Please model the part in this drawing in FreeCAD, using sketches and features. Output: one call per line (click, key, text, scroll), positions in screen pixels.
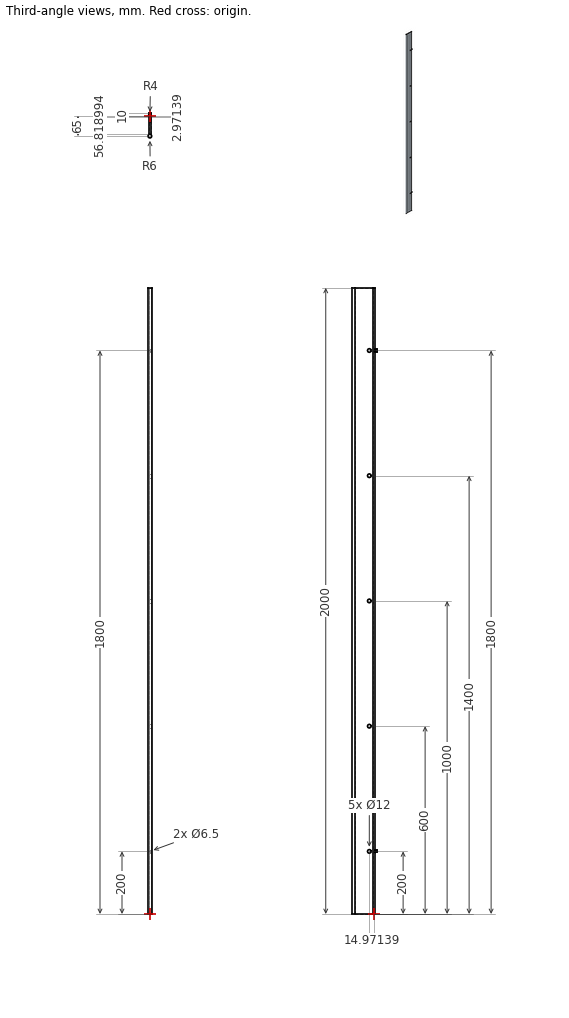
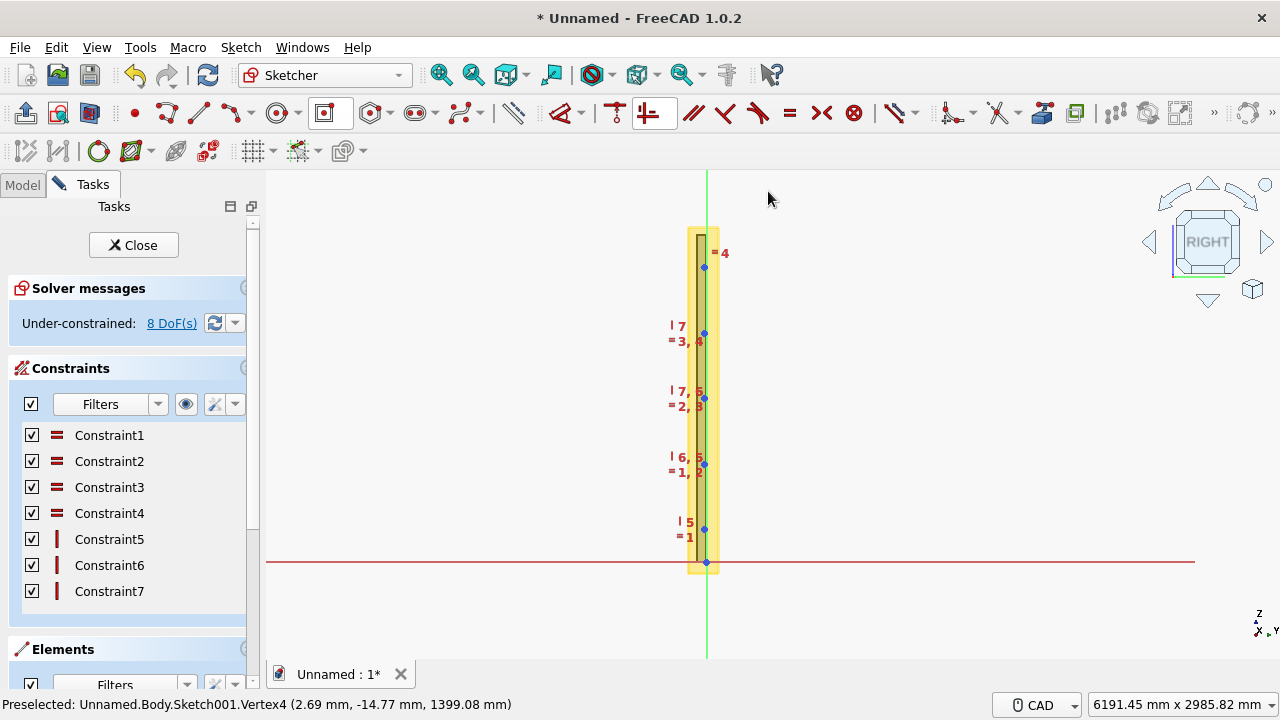
click(705, 333)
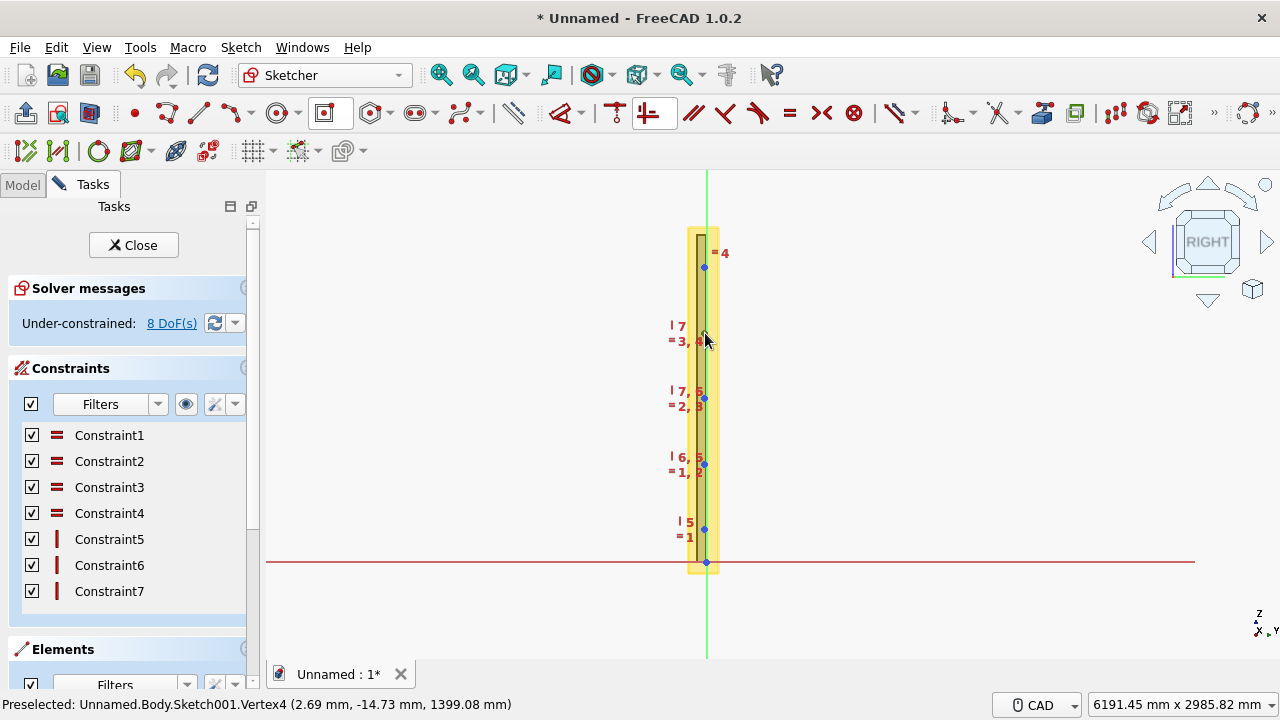
click(705, 268)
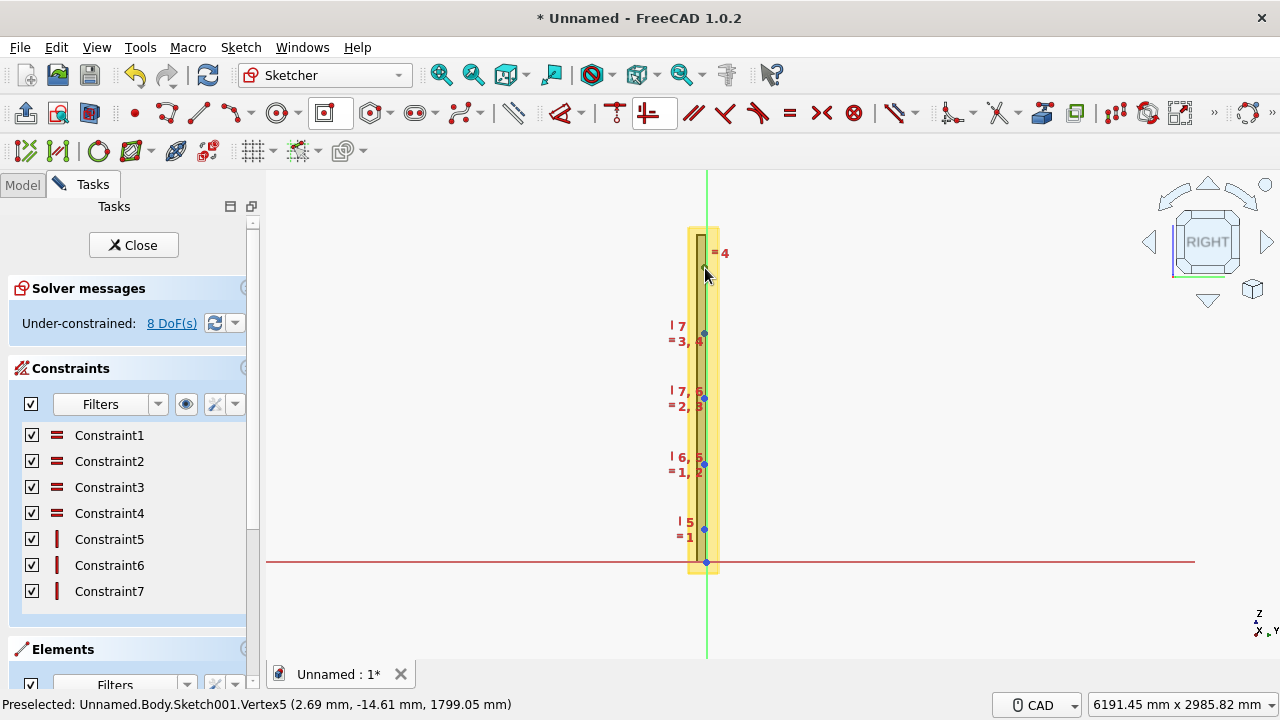
click(672, 114)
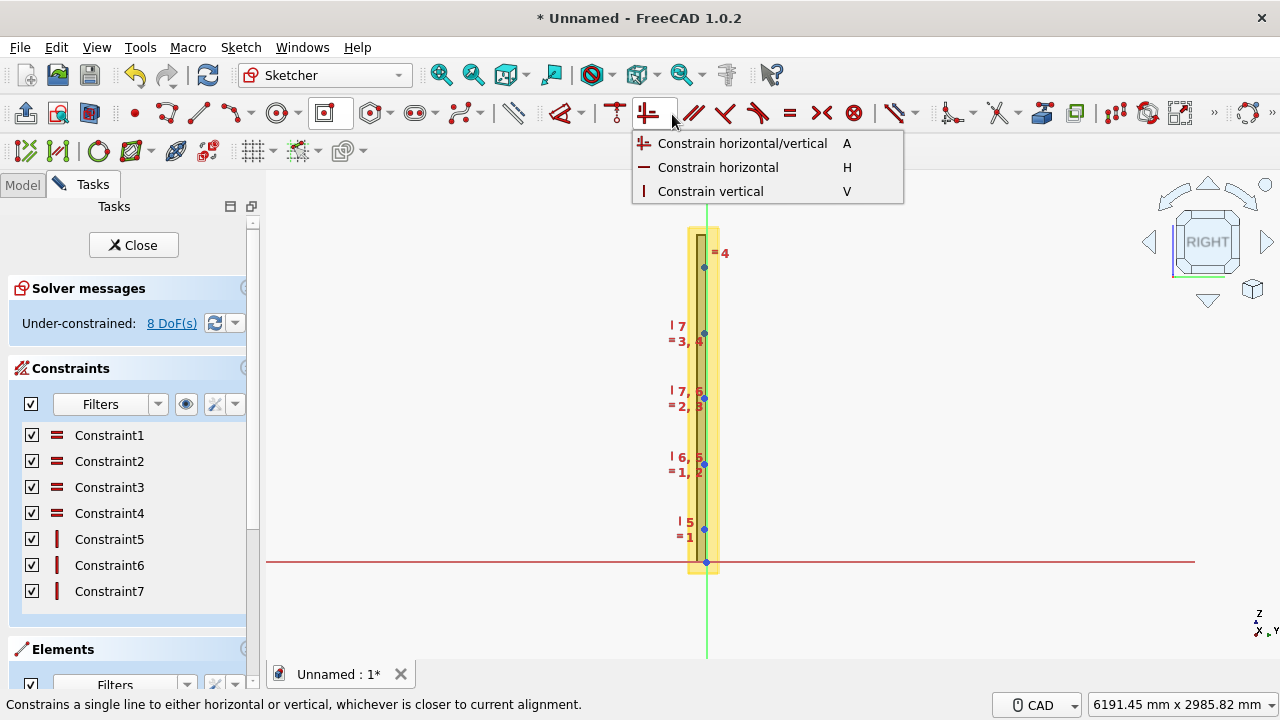
click(768, 191)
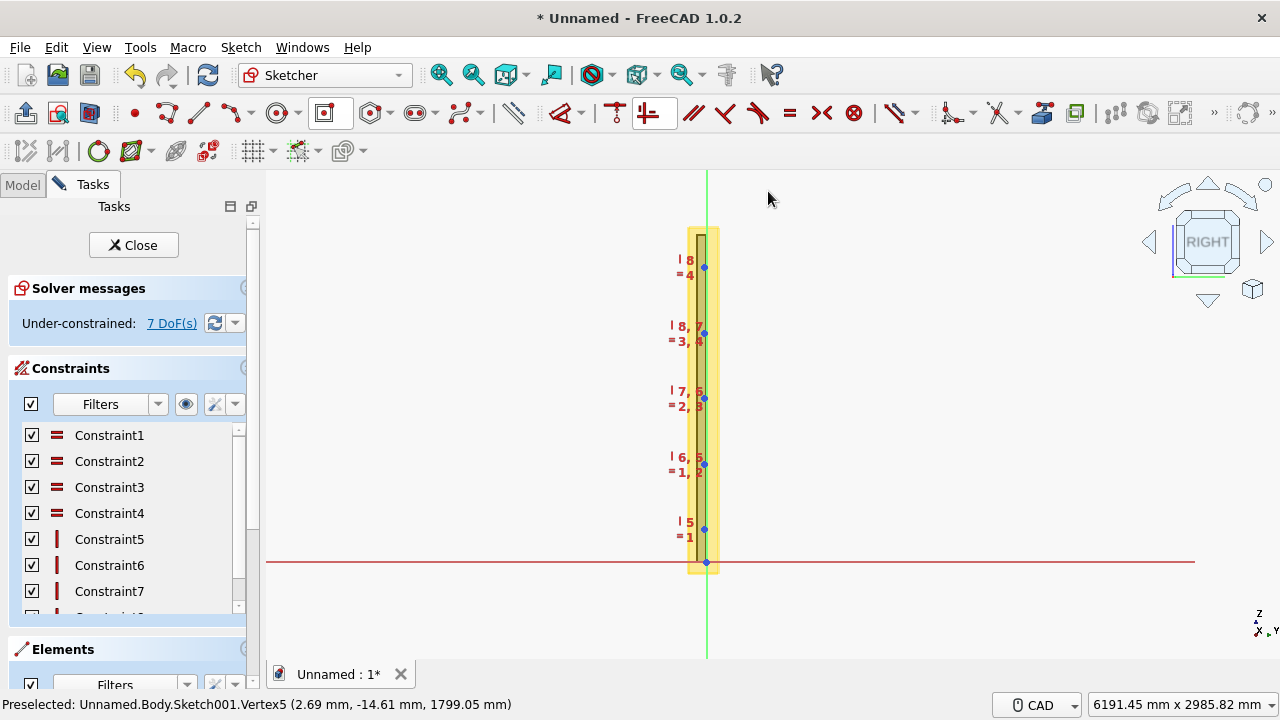
key(d)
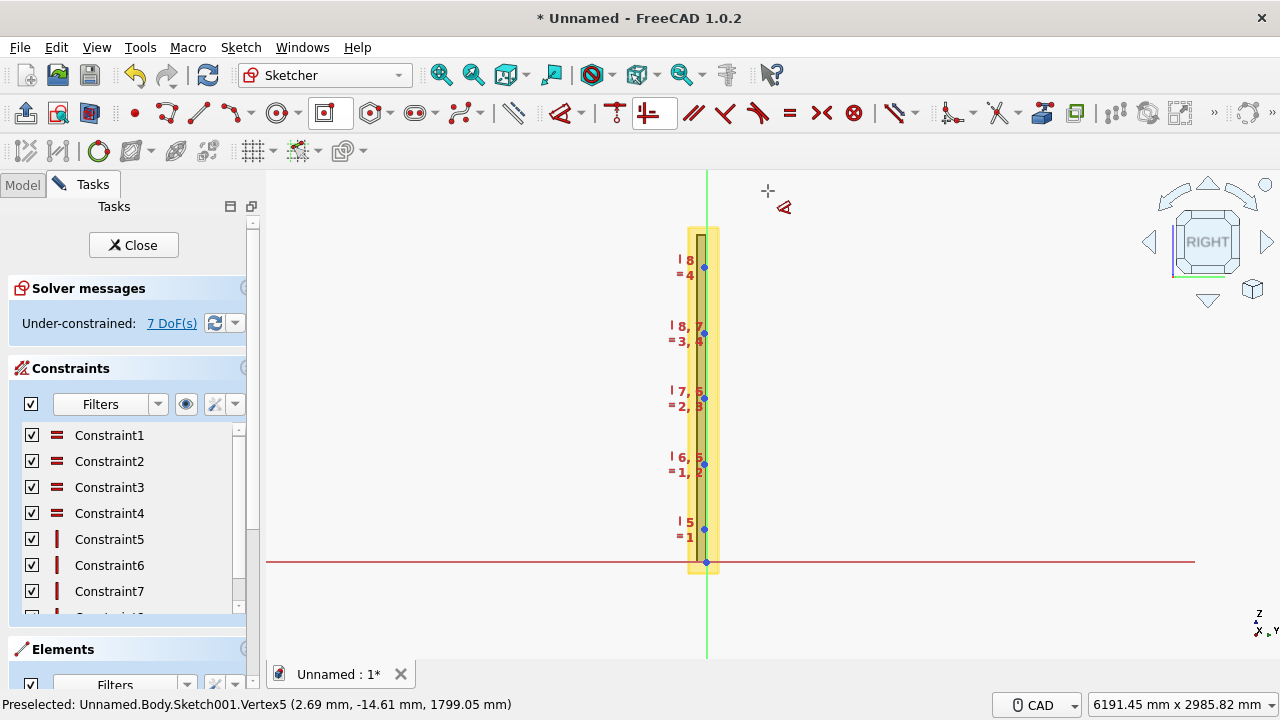
scroll(705, 529, up, 16)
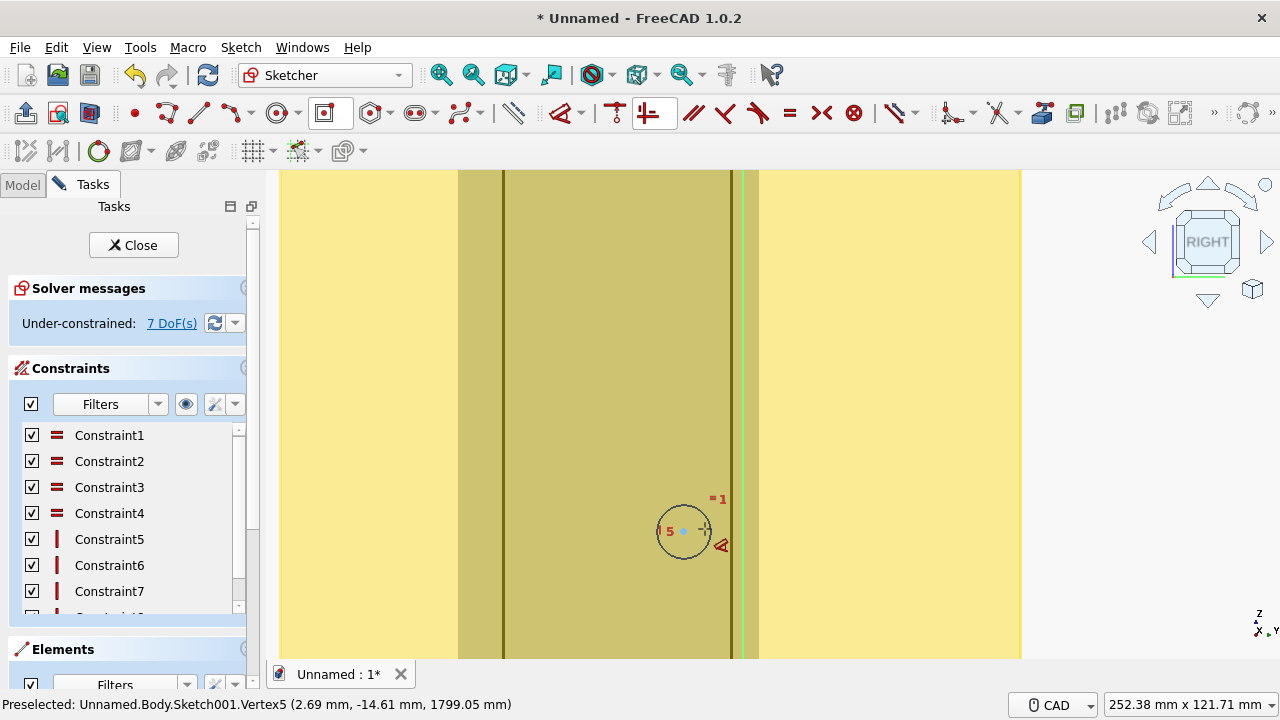
click(703, 513)
click(726, 490)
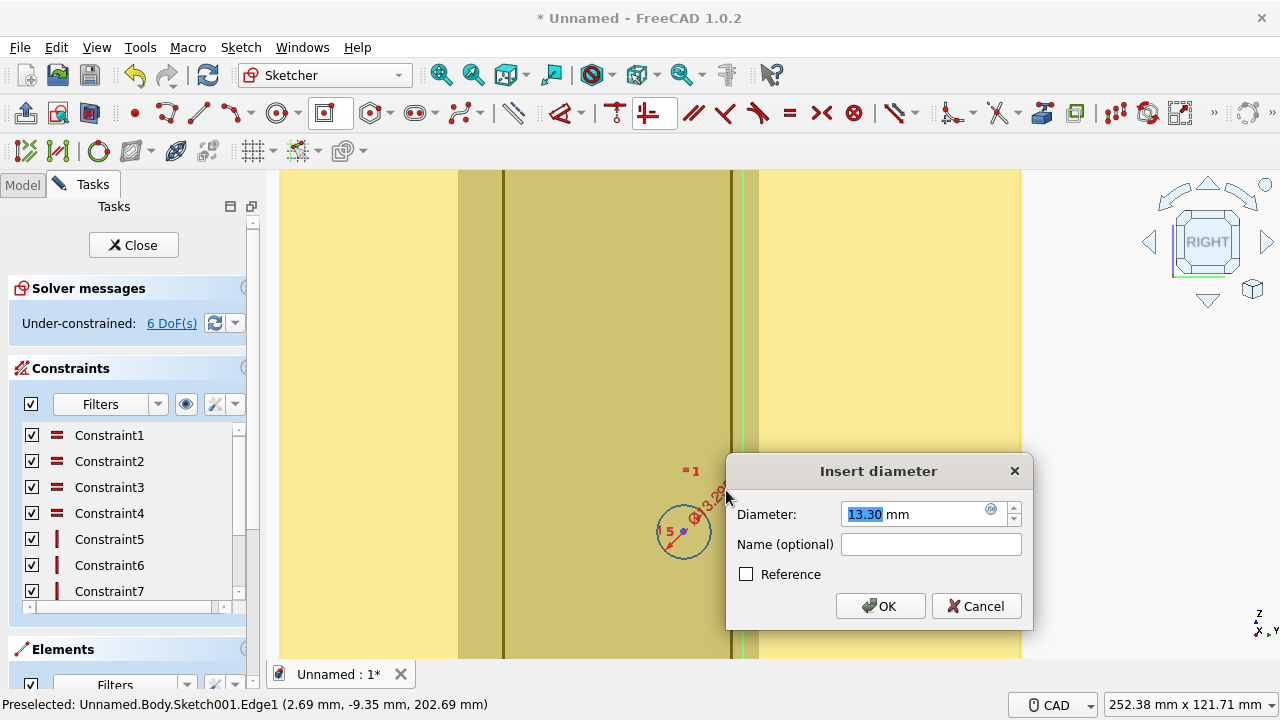
text(12)
key(Return)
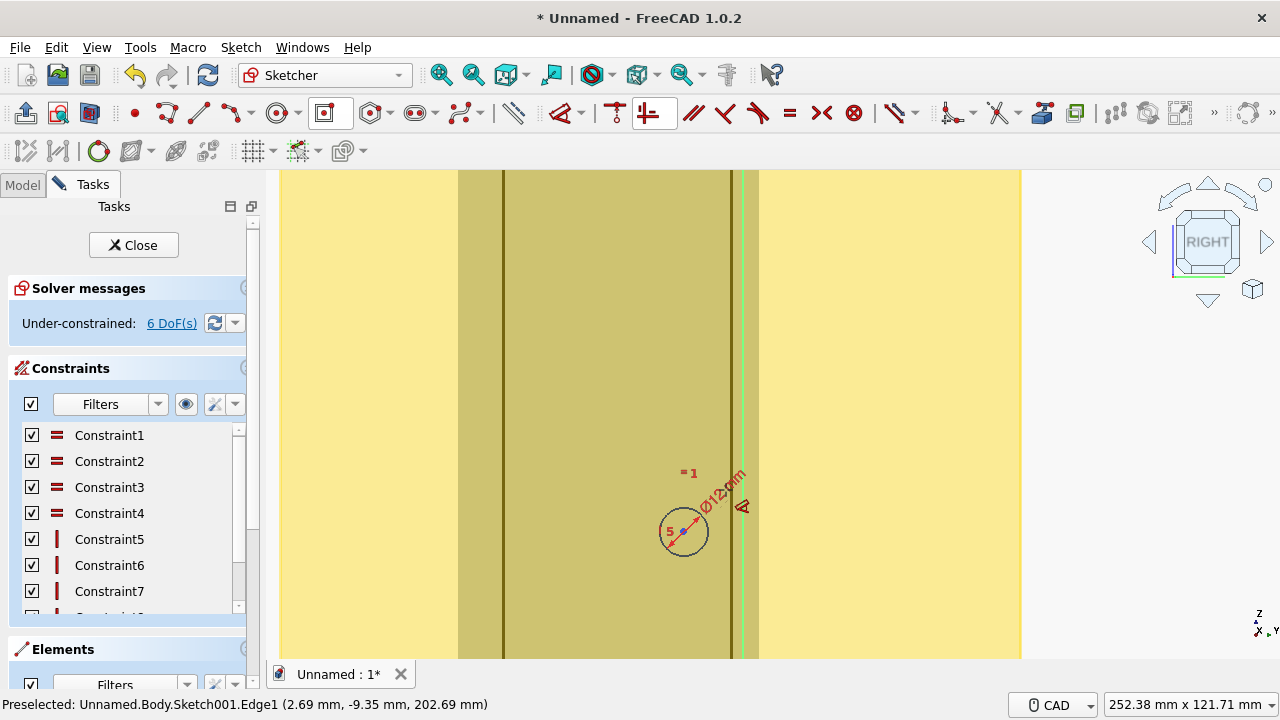
scroll(705, 557, down, 15)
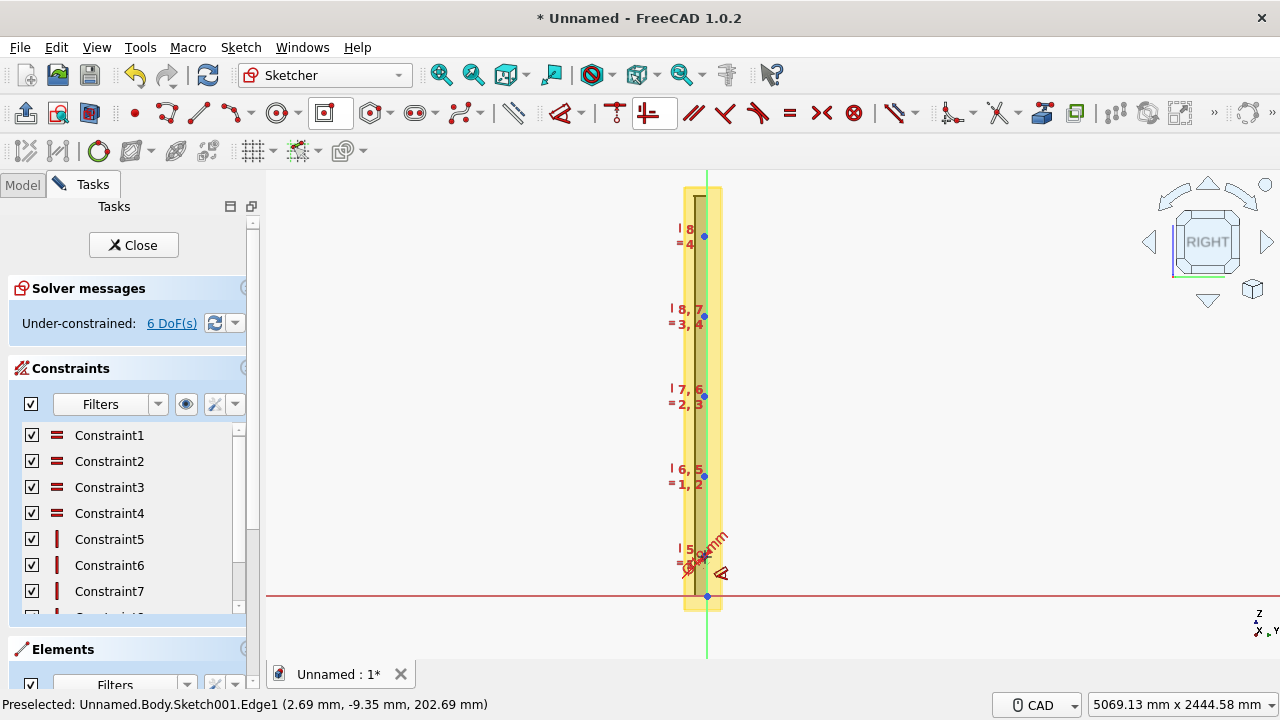
click(704, 557)
click(741, 576)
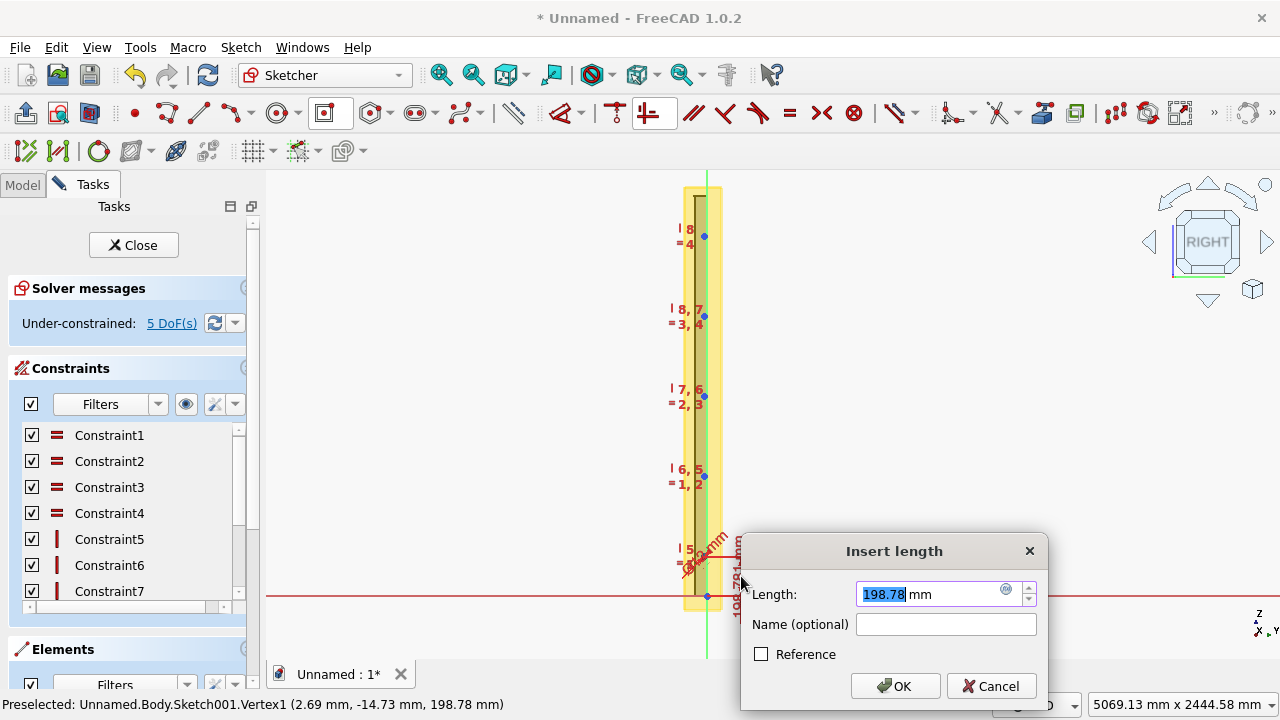
text(200)
key(Return)